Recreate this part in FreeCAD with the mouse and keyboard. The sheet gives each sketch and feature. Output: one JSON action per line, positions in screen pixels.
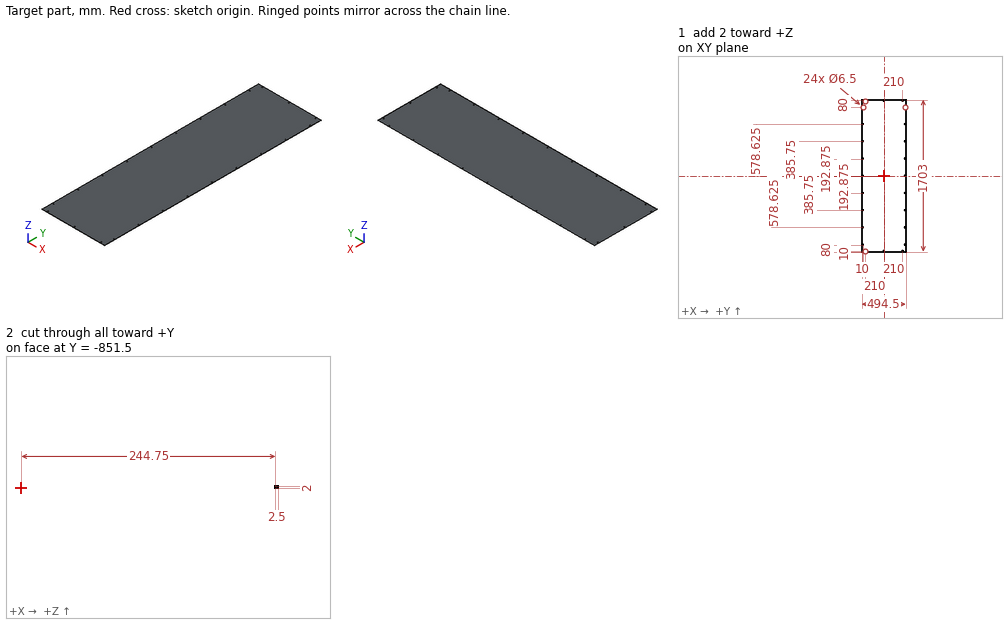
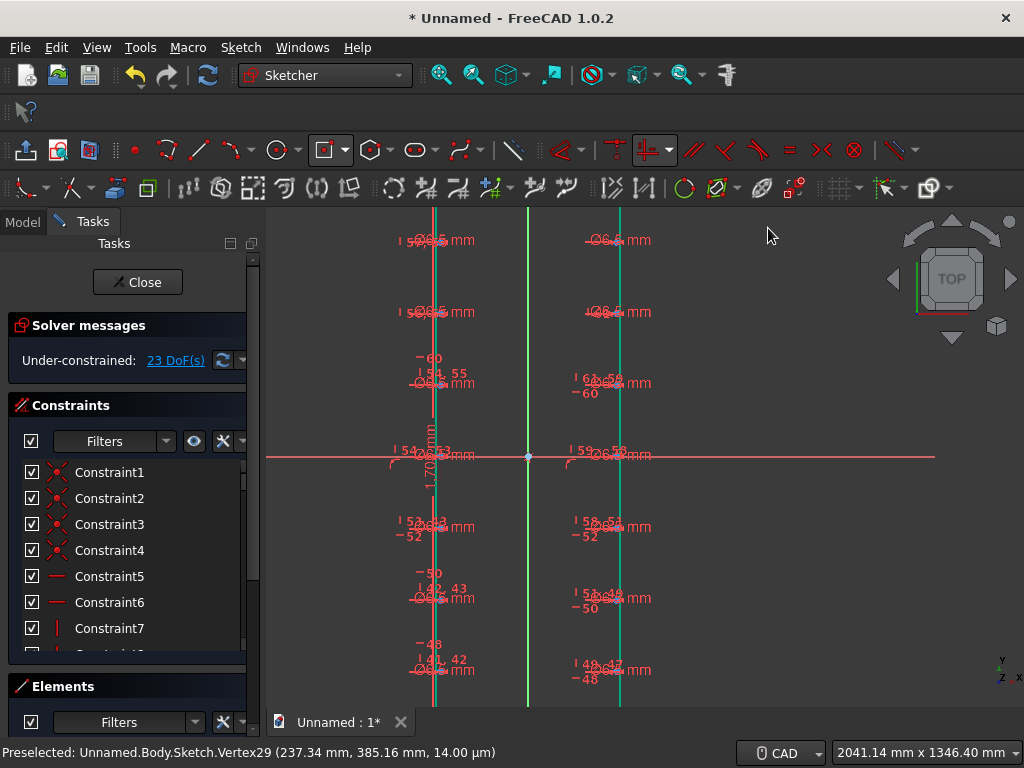
{"action": "left_click", "coordinate": [440, 314]}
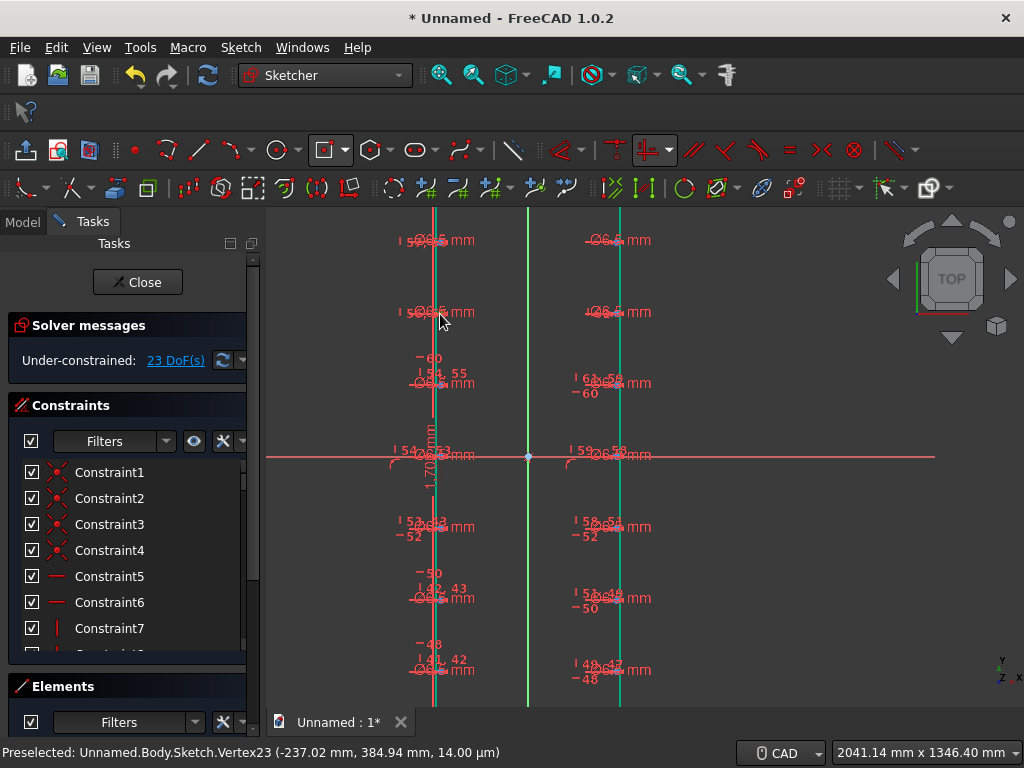
{"action": "left_click", "coordinate": [616, 314]}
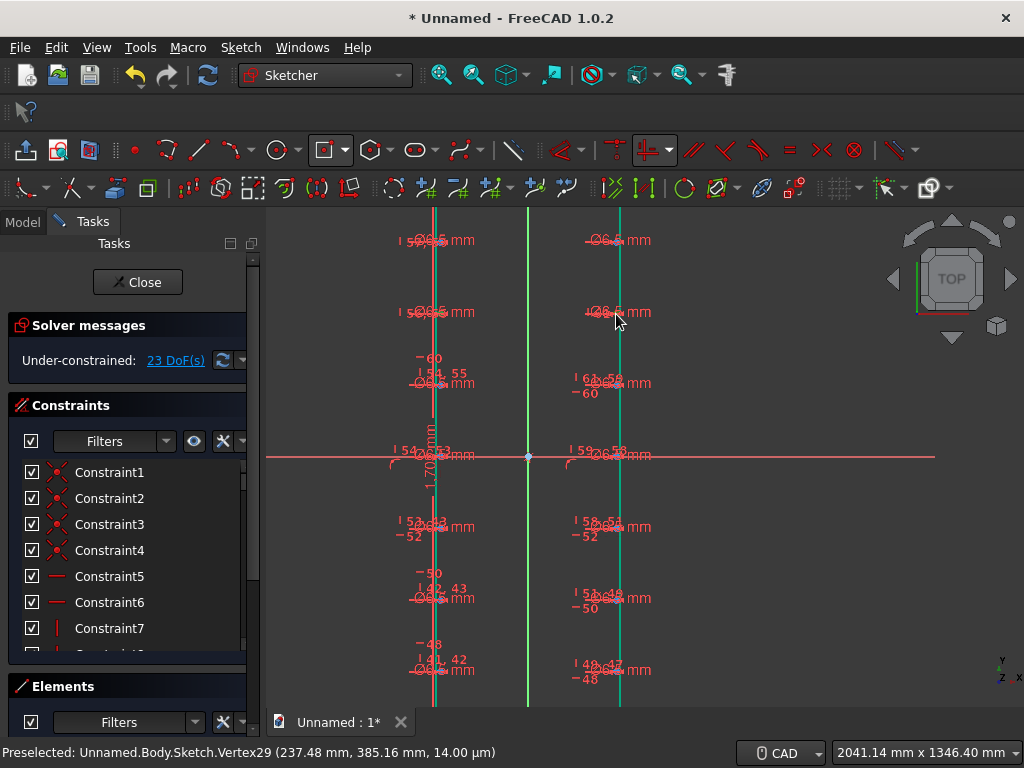
{"action": "key", "text": "h"}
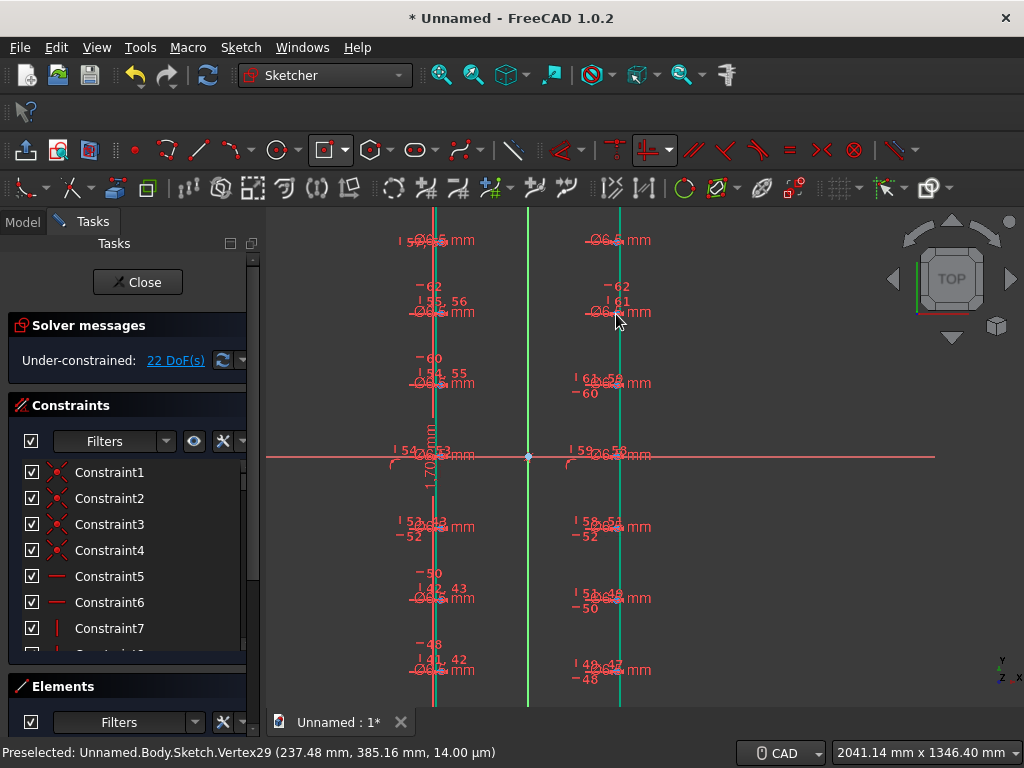
{"action": "scroll", "coordinate": [616, 457], "scroll_direction": "down", "scroll_amount": 4}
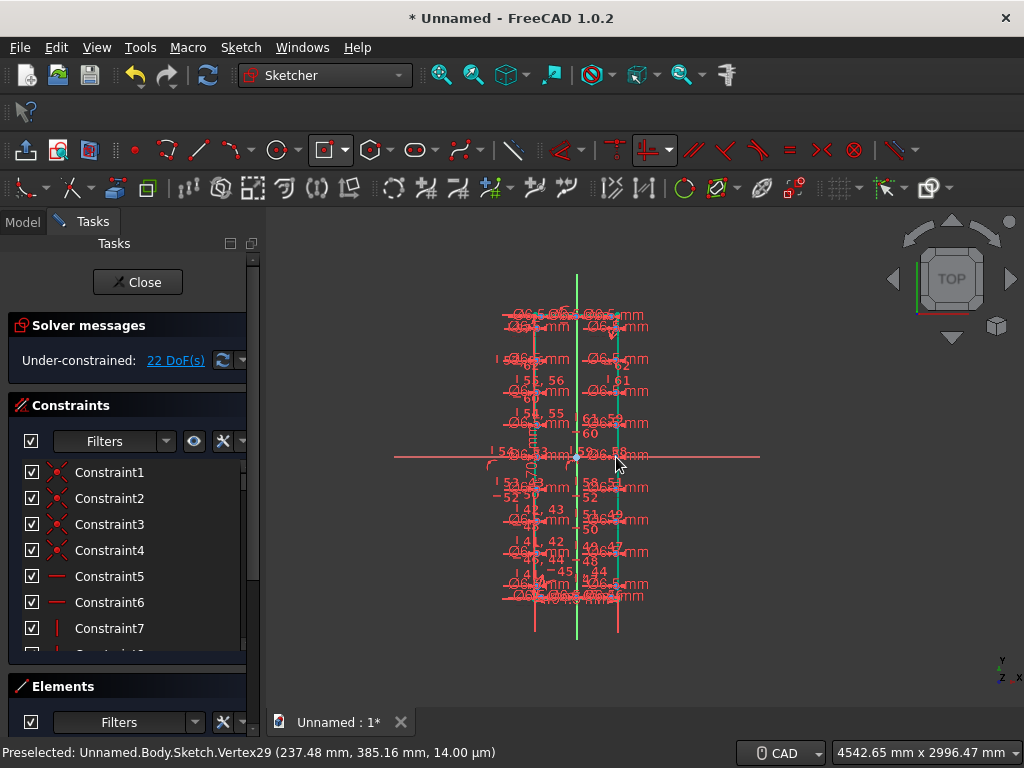
{"action": "scroll", "coordinate": [542, 317], "scroll_direction": "up", "scroll_amount": 4}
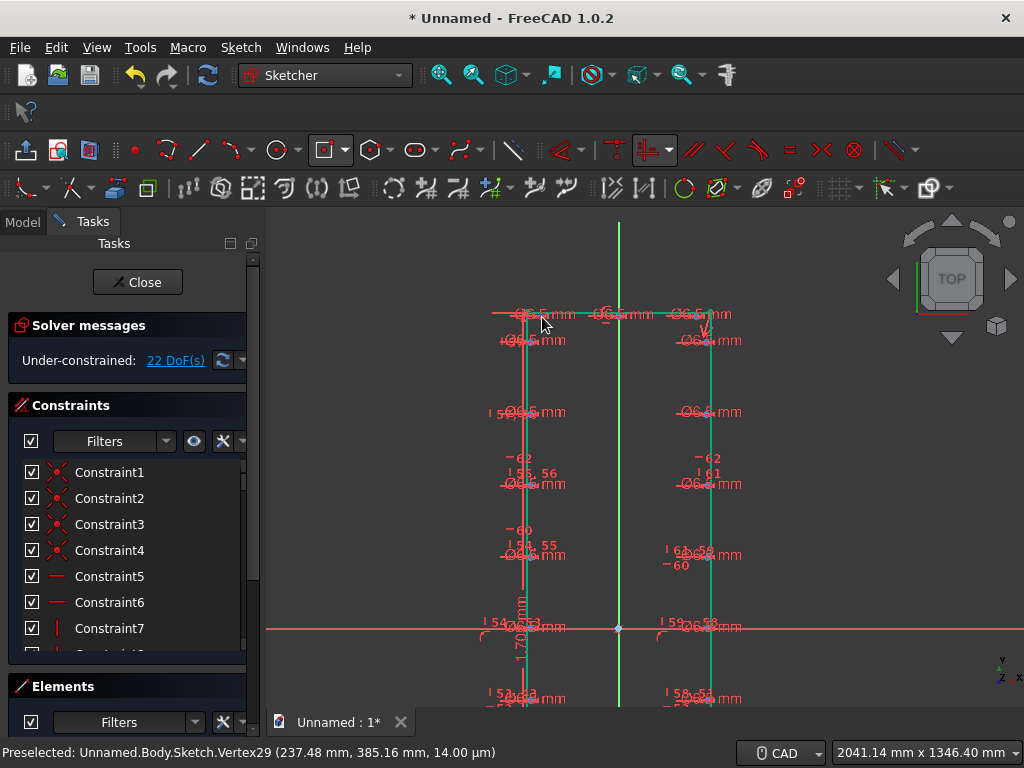
{"action": "left_click", "coordinate": [541, 316]}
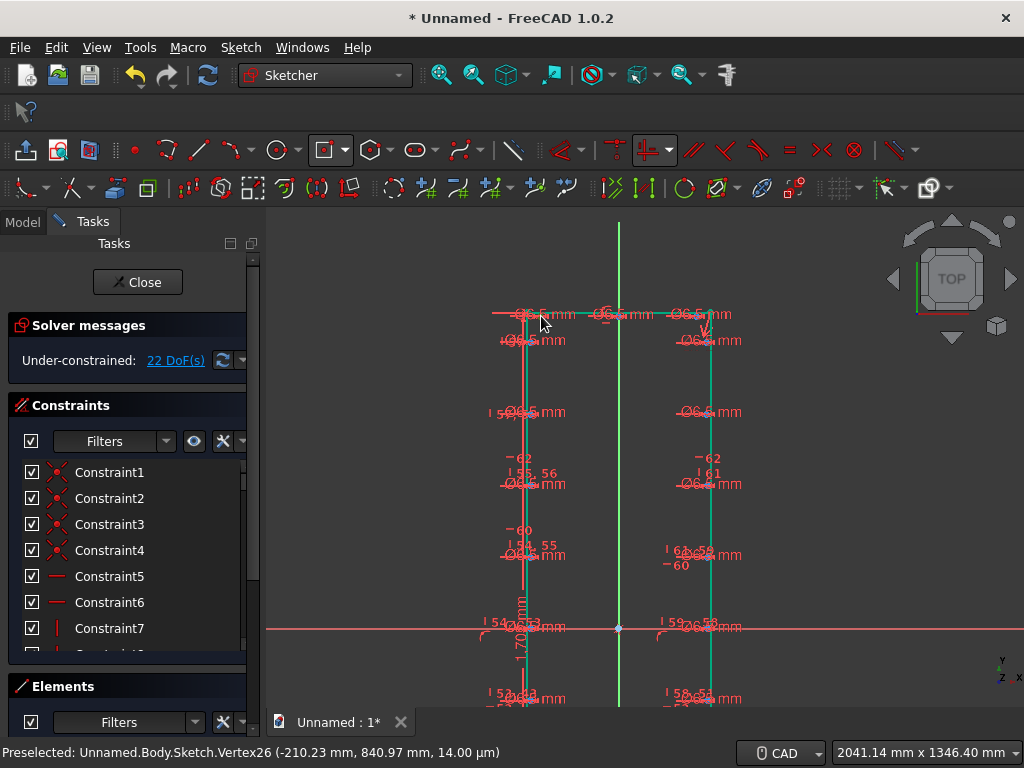
{"action": "left_click", "coordinate": [619, 316]}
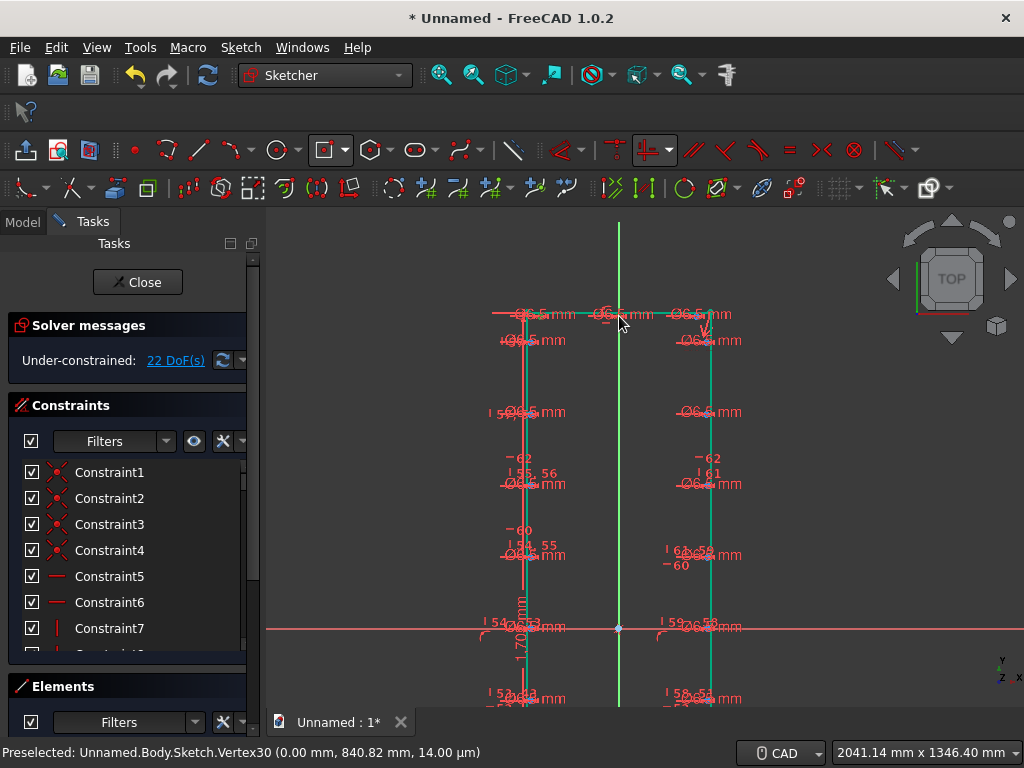
{"action": "left_click", "coordinate": [672, 150]}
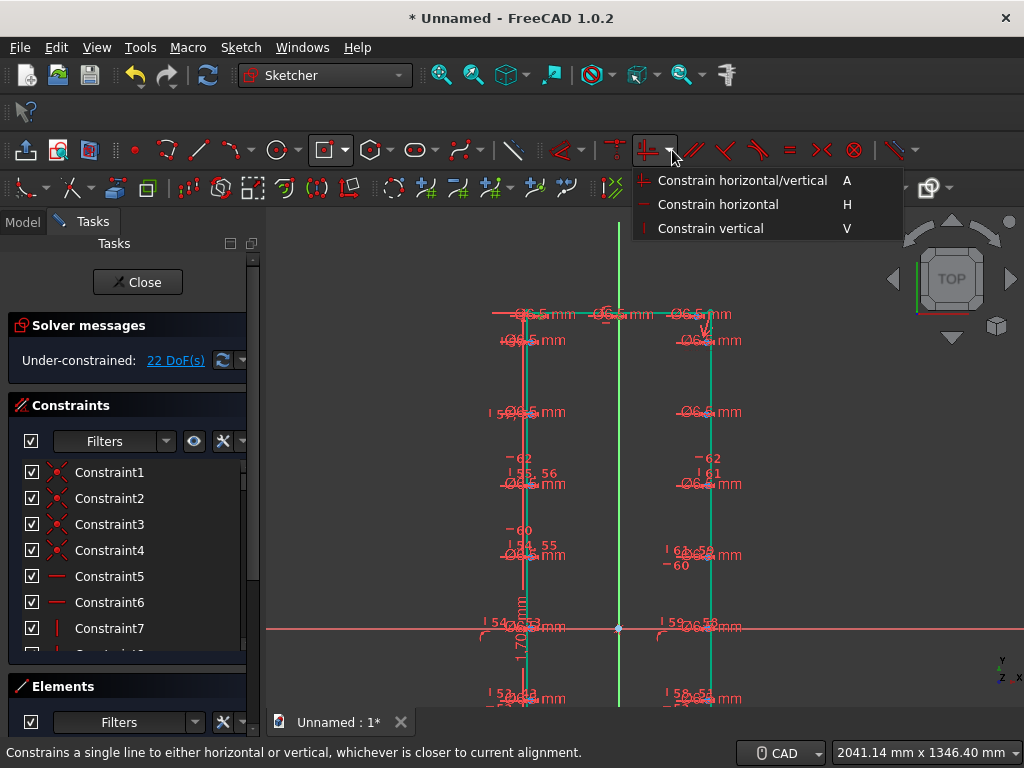
{"action": "left_click", "coordinate": [768, 204]}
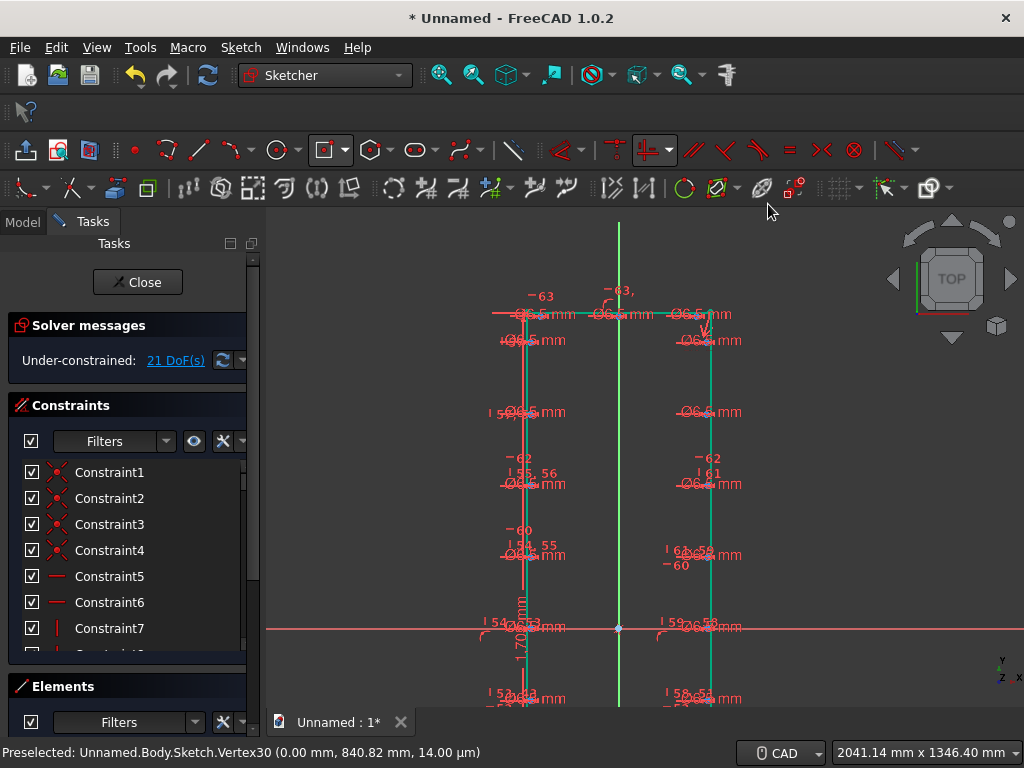
{"action": "left_click", "coordinate": [707, 486]}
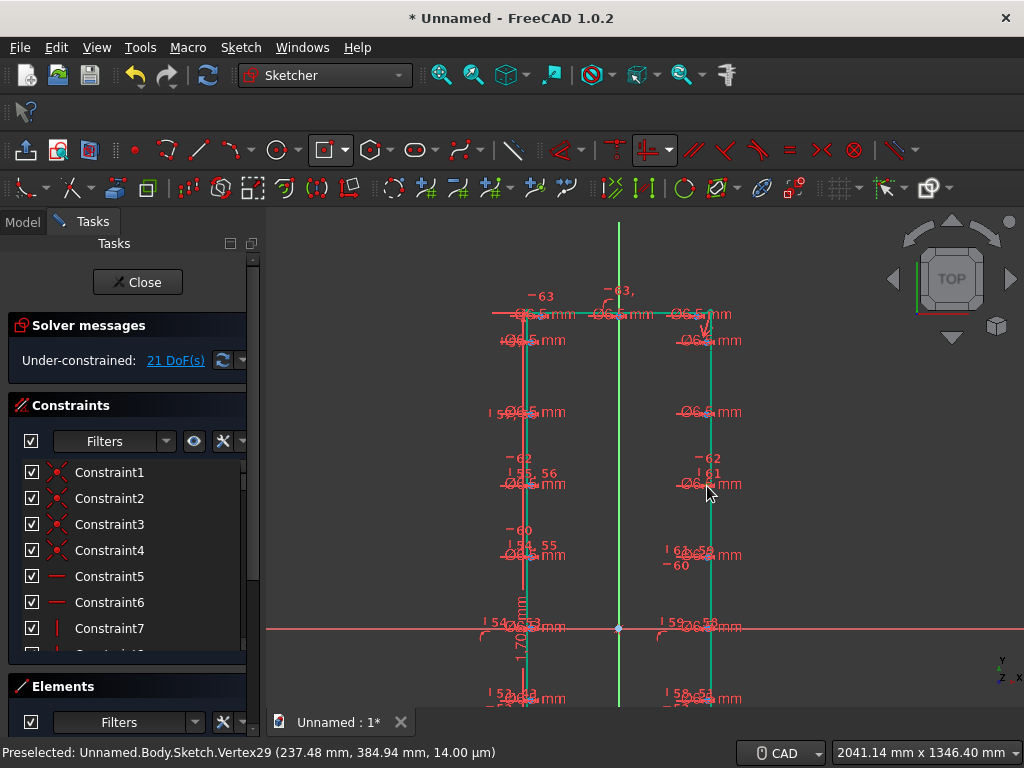
{"action": "left_click", "coordinate": [707, 414]}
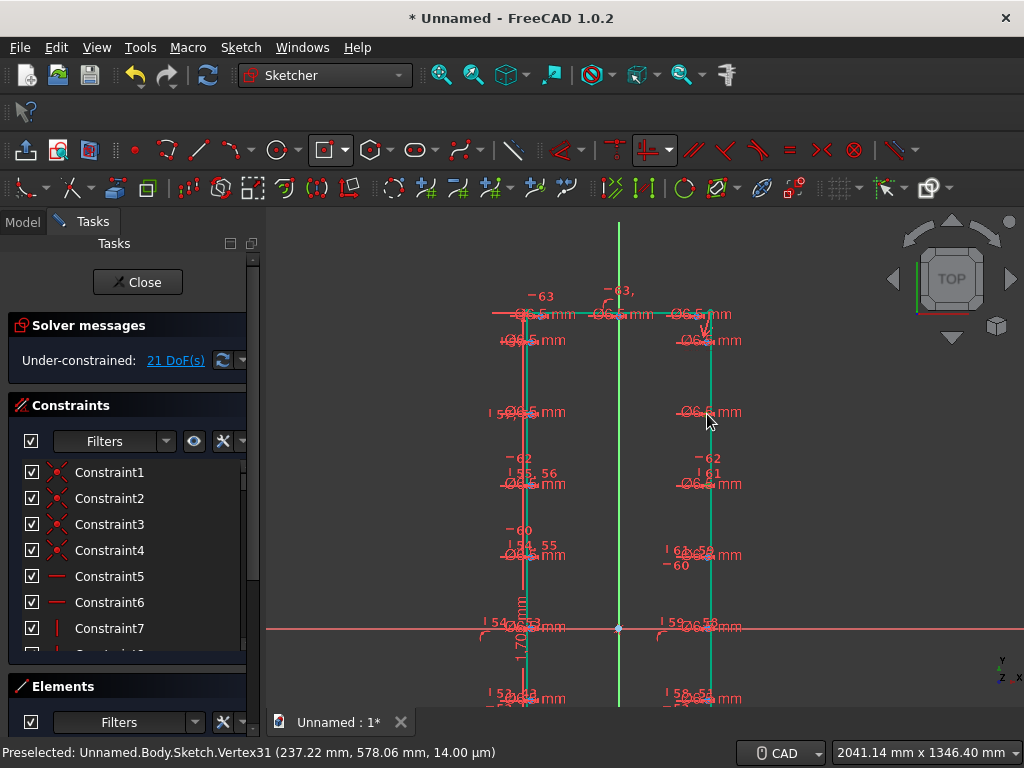
{"action": "key", "text": "v"}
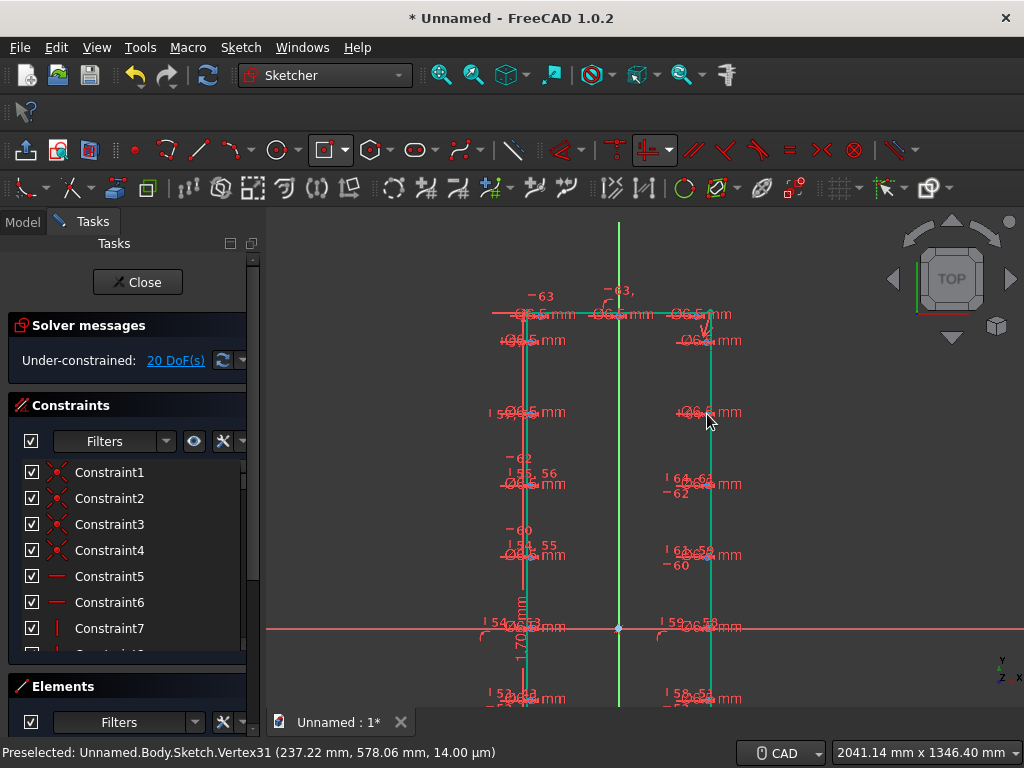
{"action": "left_click", "coordinate": [531, 414]}